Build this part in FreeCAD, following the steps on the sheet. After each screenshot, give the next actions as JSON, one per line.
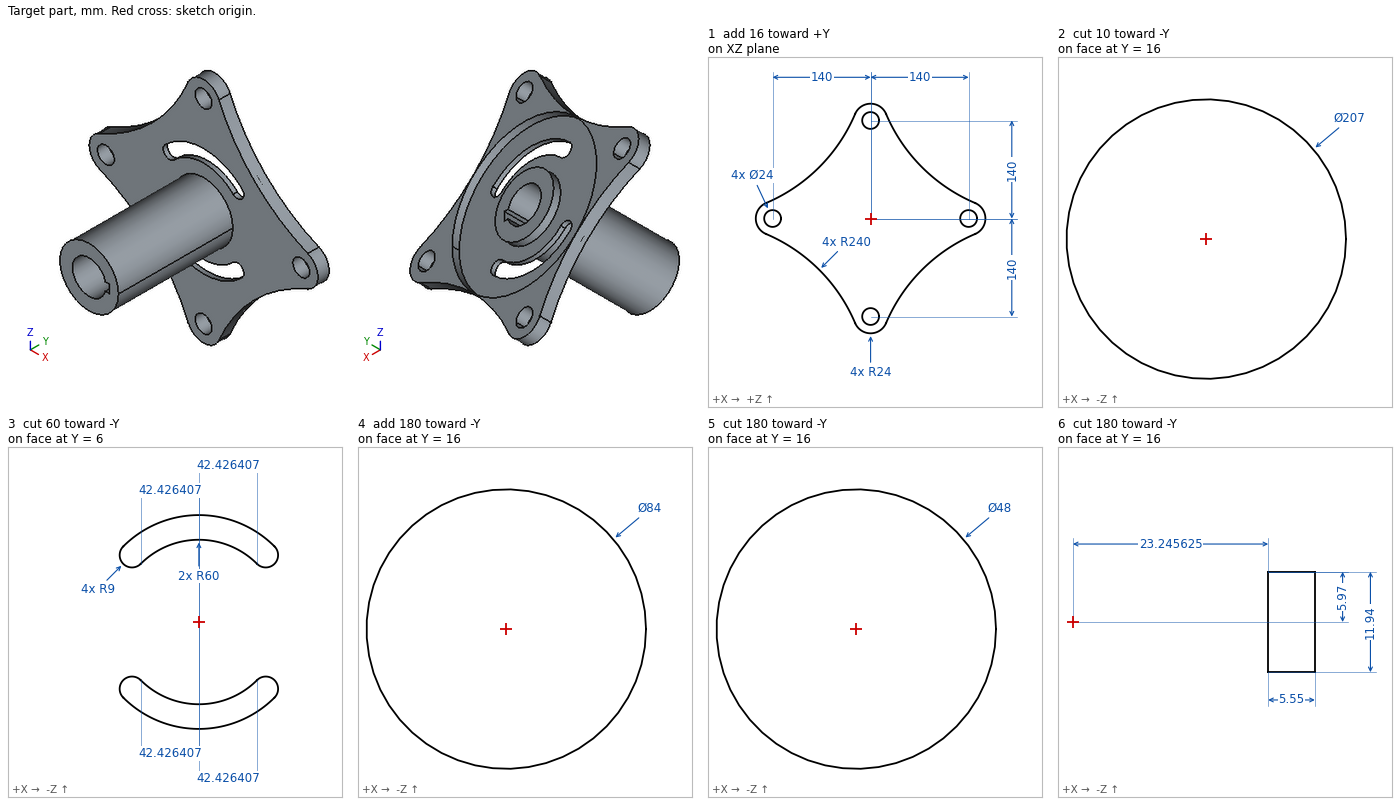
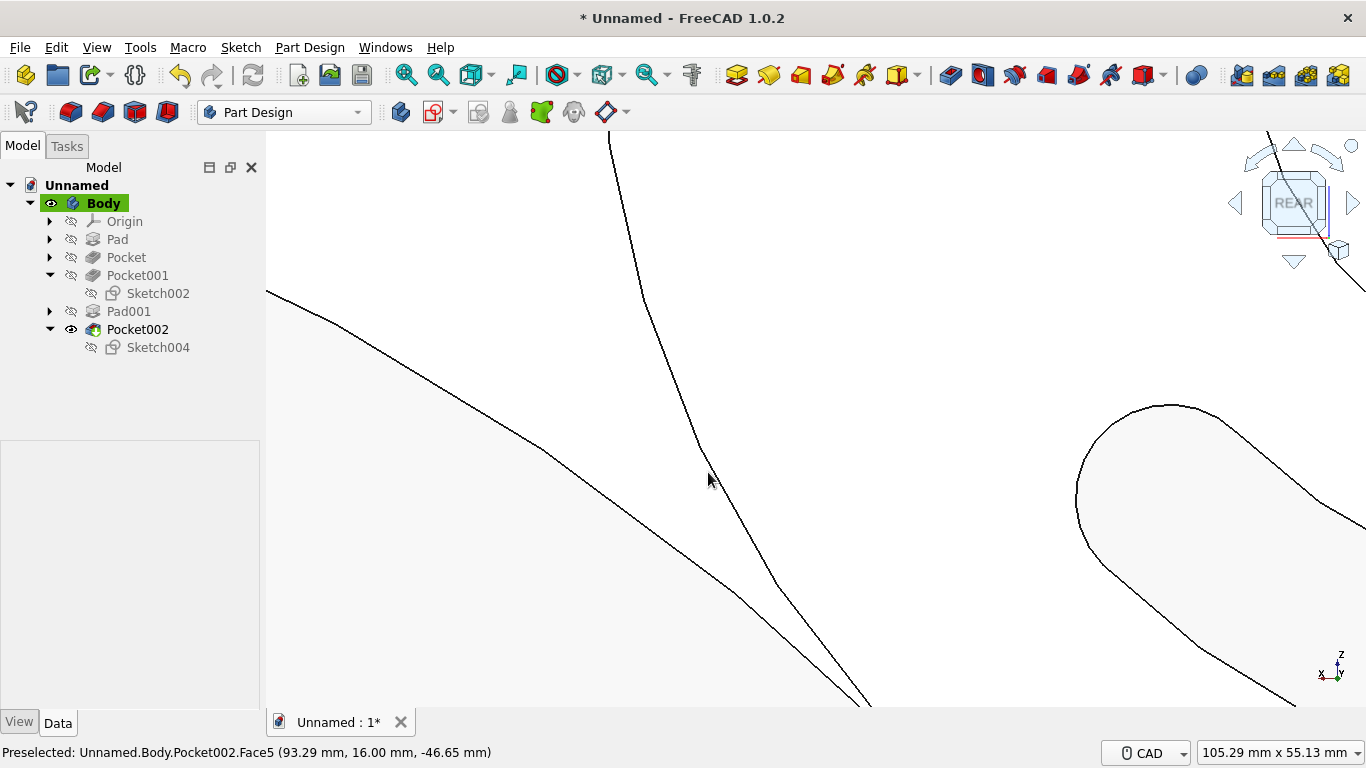
{"action": "left_click", "coordinate": [700, 477]}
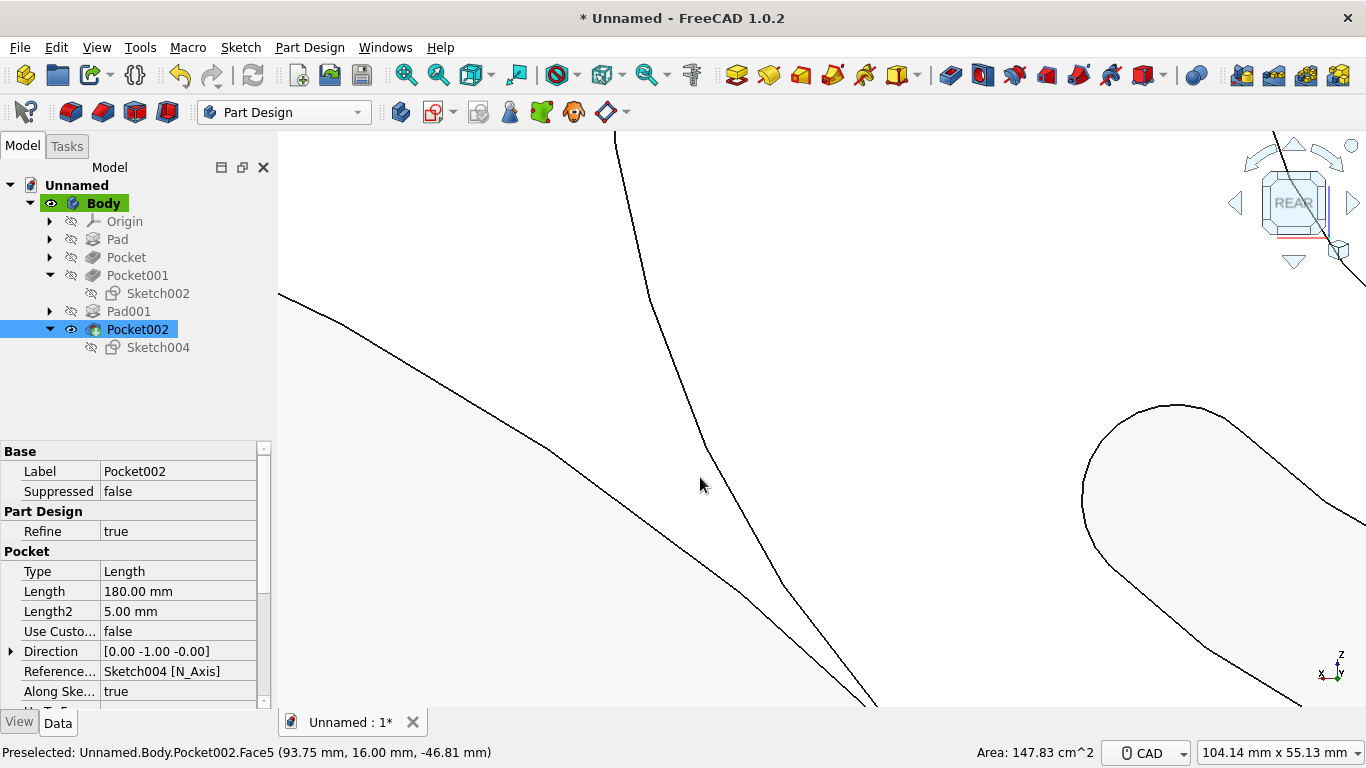
{"action": "left_click", "coordinate": [434, 112]}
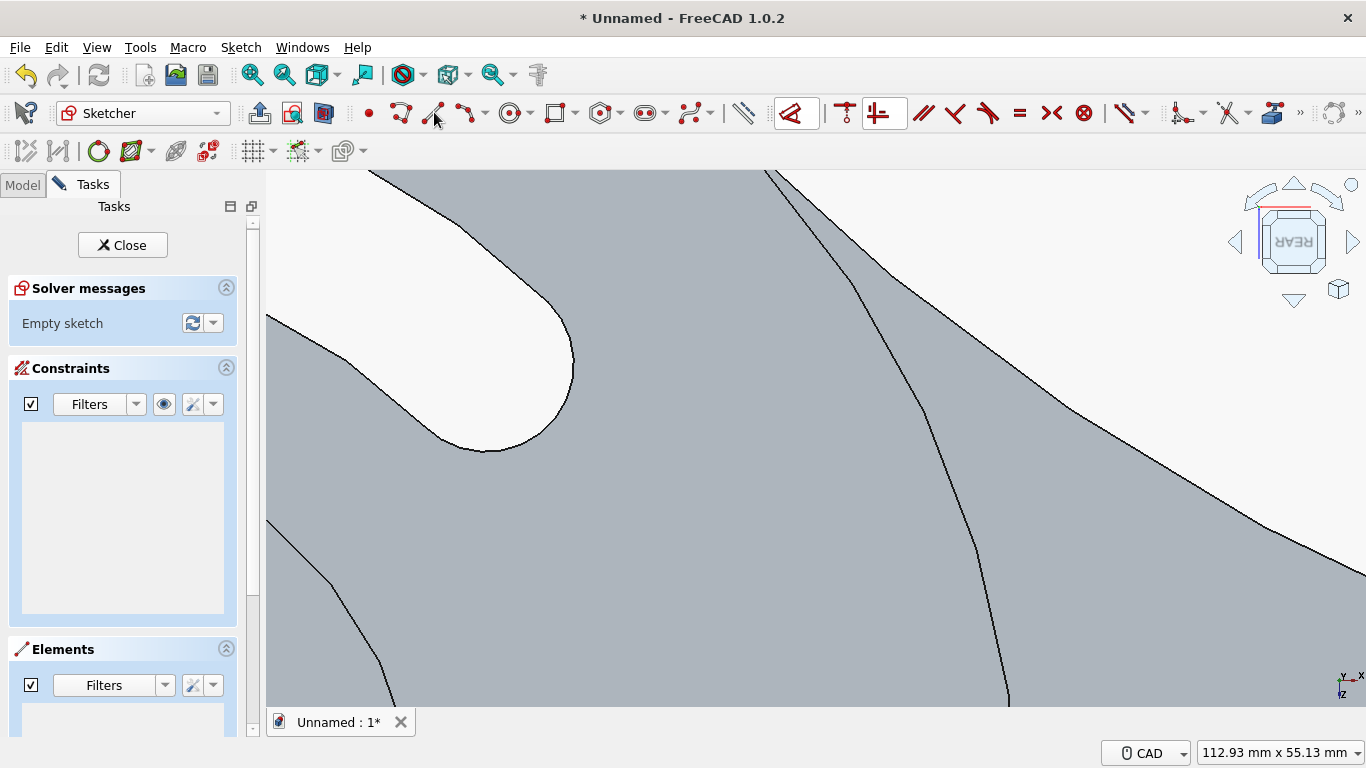
{"action": "scroll", "coordinate": [748, 438], "scroll_direction": "down", "scroll_amount": 5}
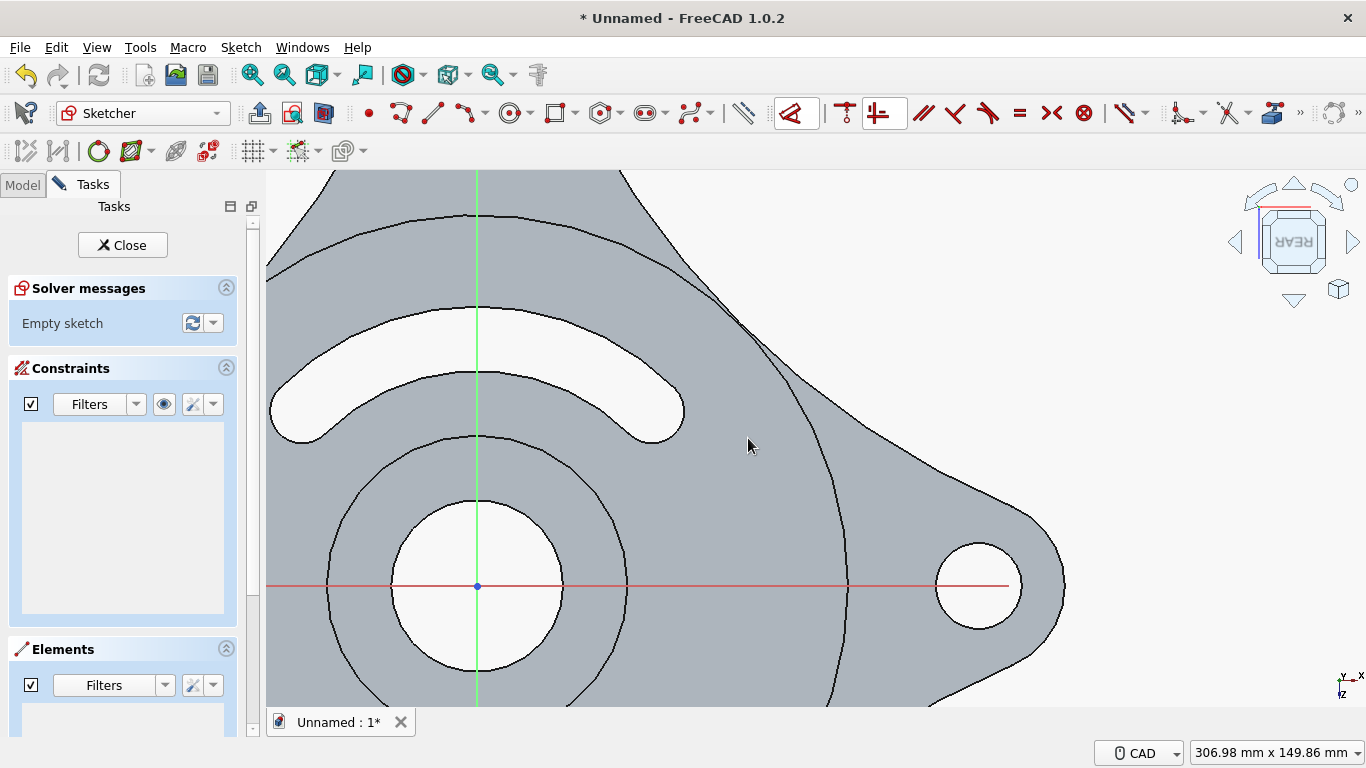
{"action": "scroll", "coordinate": [485, 615], "scroll_direction": "up", "scroll_amount": 9}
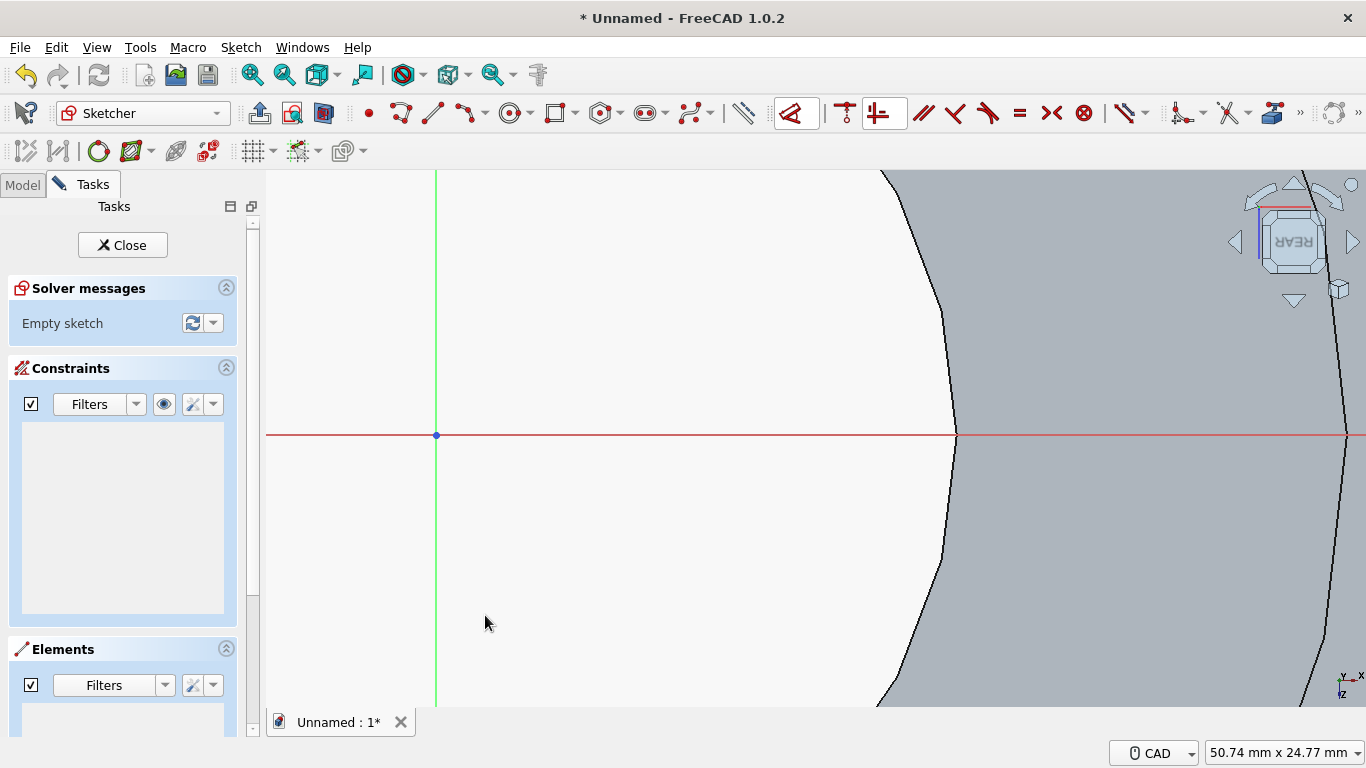
{"action": "left_click", "coordinate": [556, 114]}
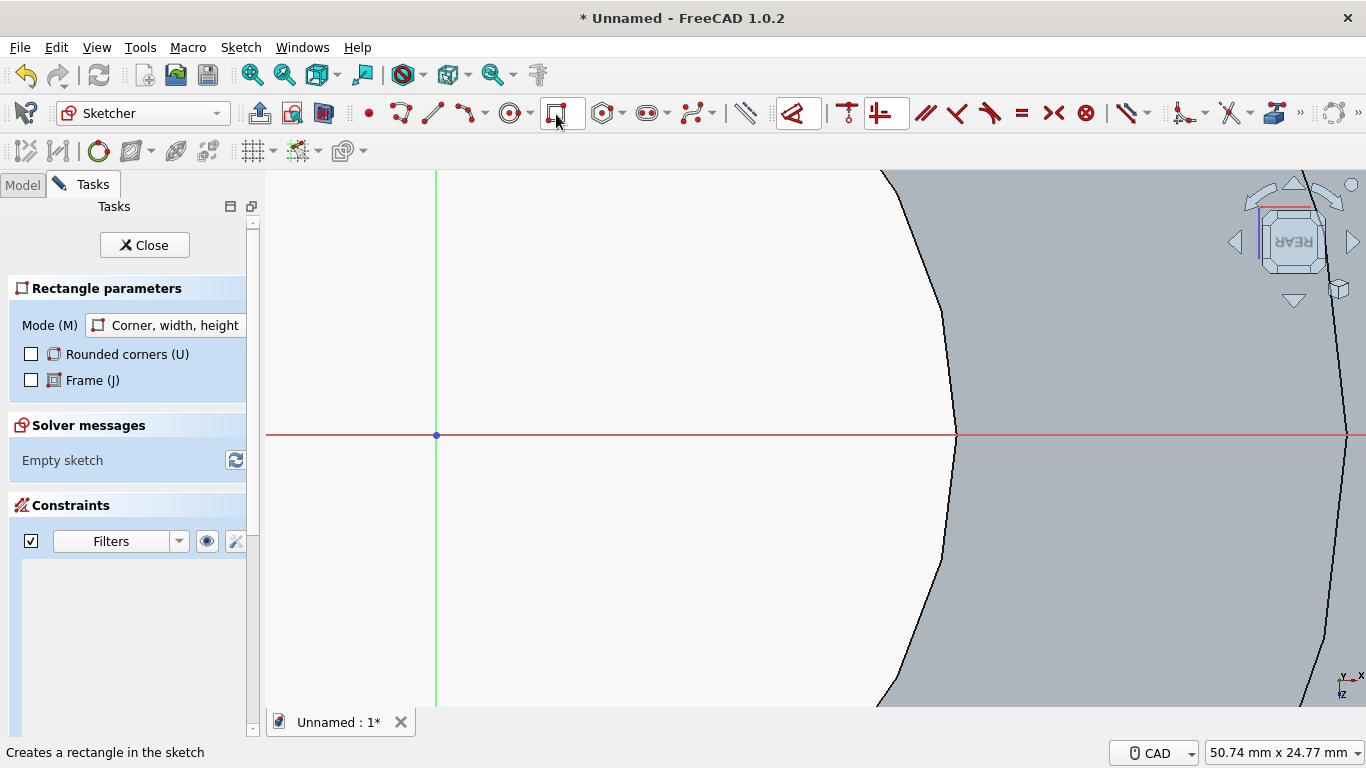
{"action": "left_click", "coordinate": [940, 306]}
{"action": "left_click", "coordinate": [1061, 565]}
{"action": "key", "text": "Escape"}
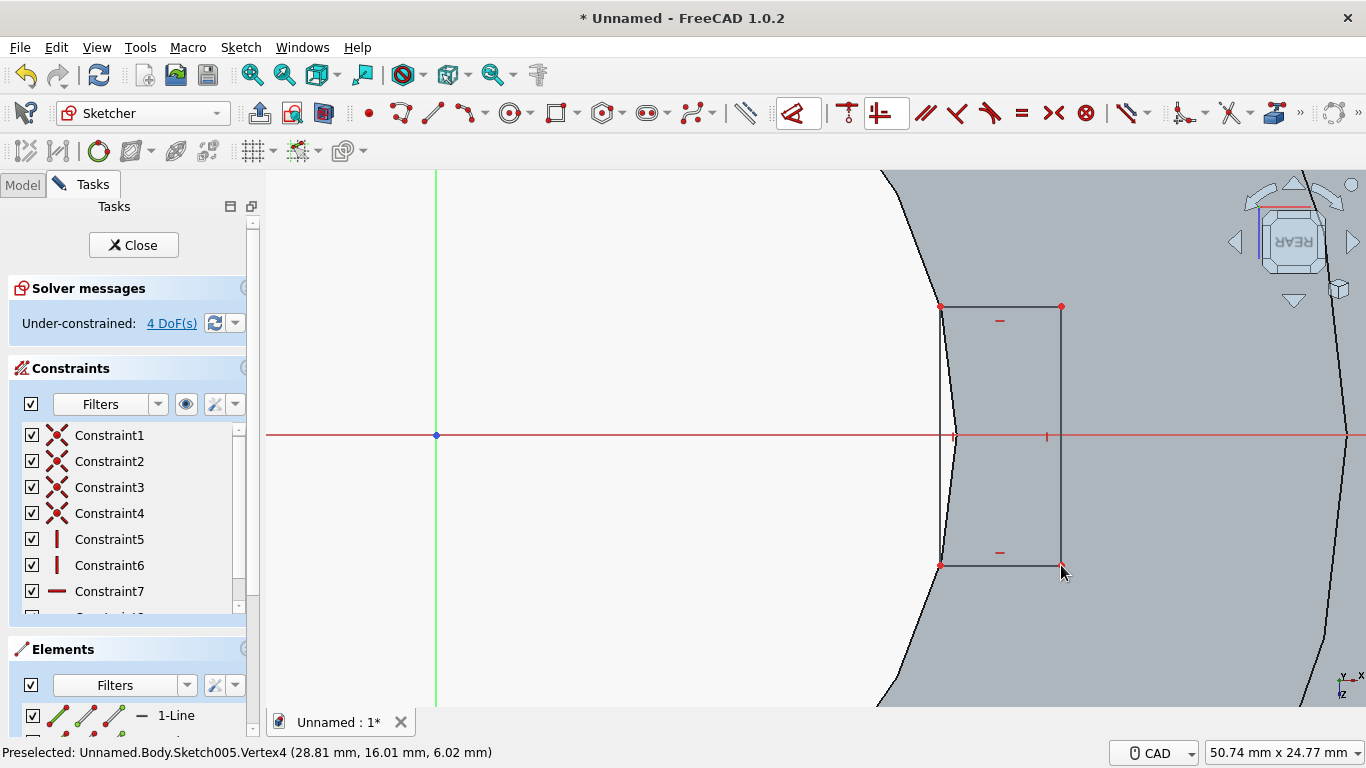
{"action": "left_click", "coordinate": [976, 566]}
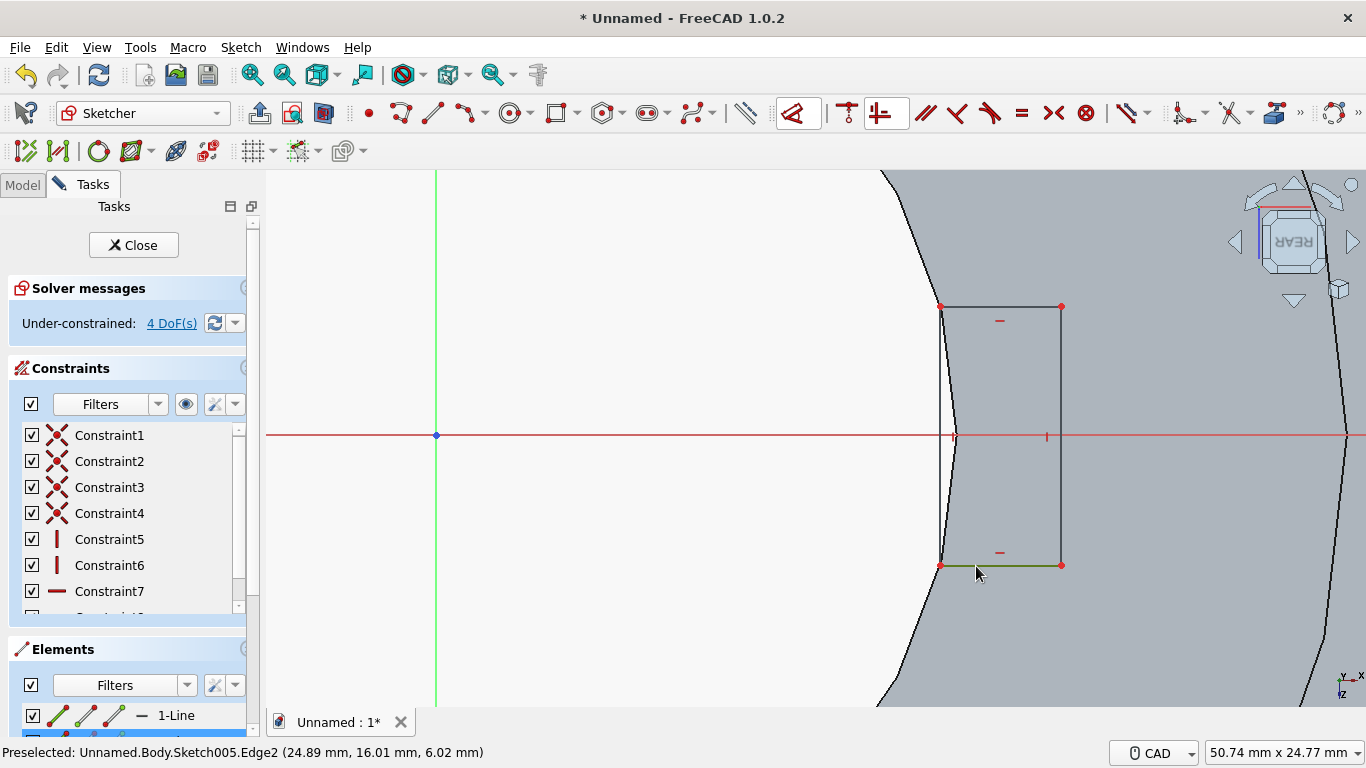
{"action": "key", "text": "l"}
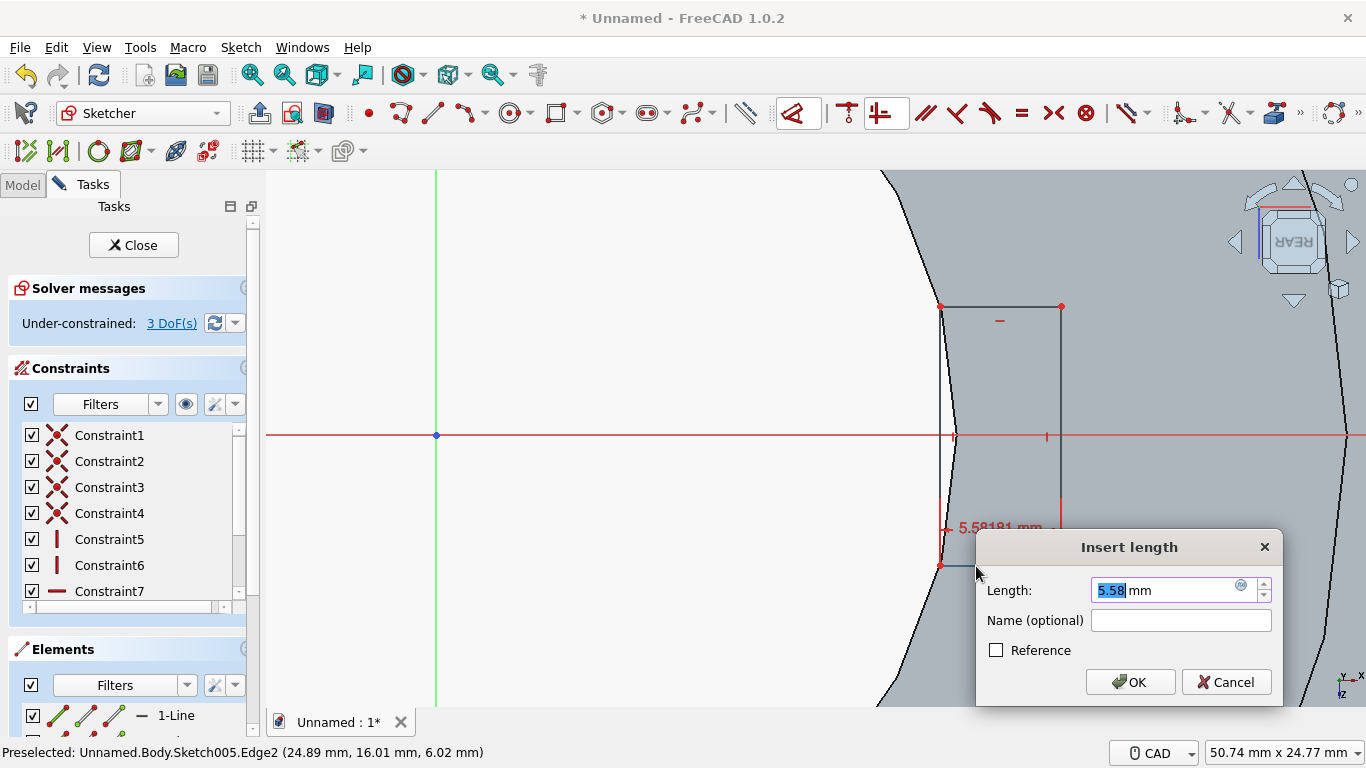
{"action": "type", "text": "5.55"}
{"action": "key", "text": "Return"}